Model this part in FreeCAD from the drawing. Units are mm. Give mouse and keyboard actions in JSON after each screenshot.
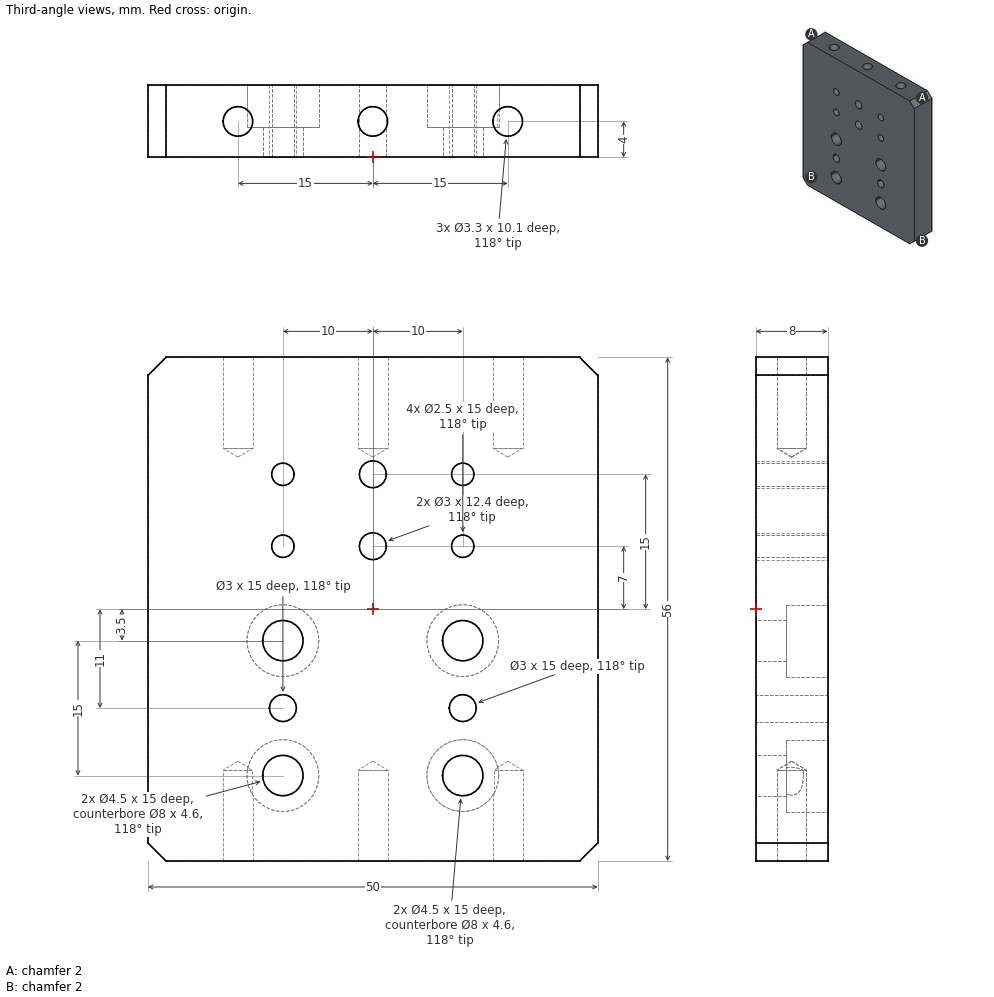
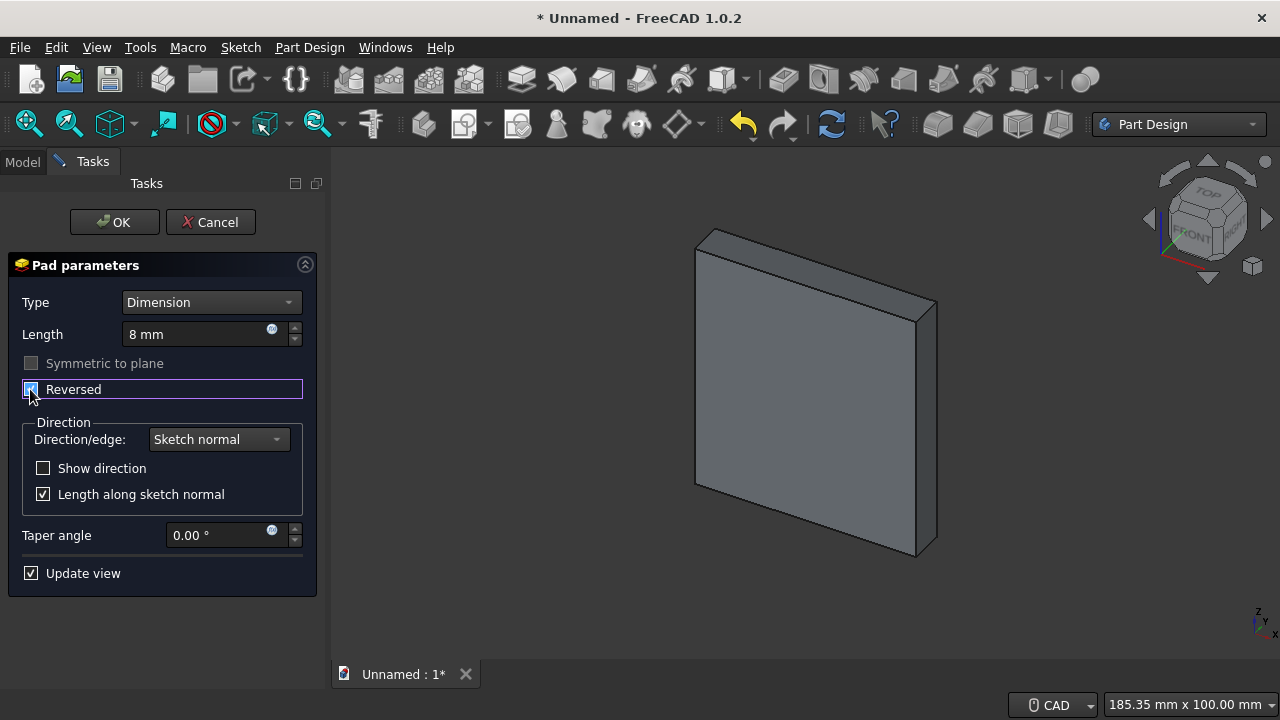
{"action": "left_click", "coordinate": [115, 222]}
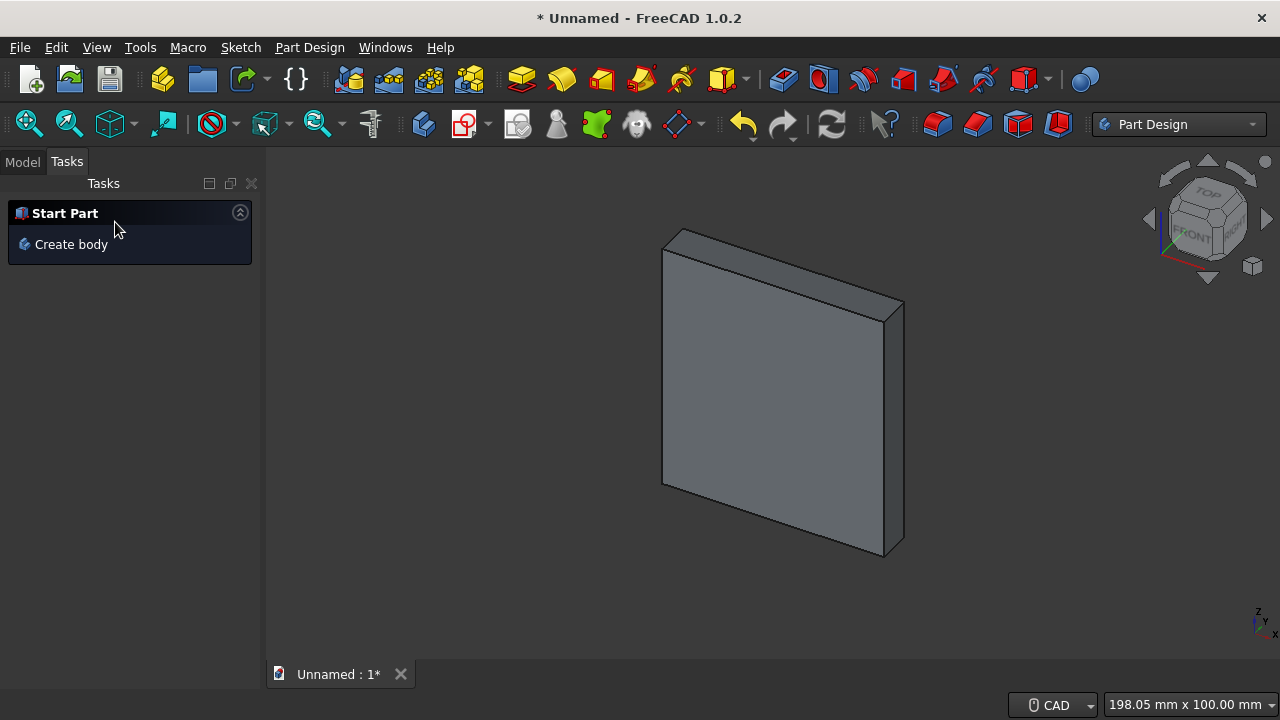
{"action": "left_click", "coordinate": [847, 295]}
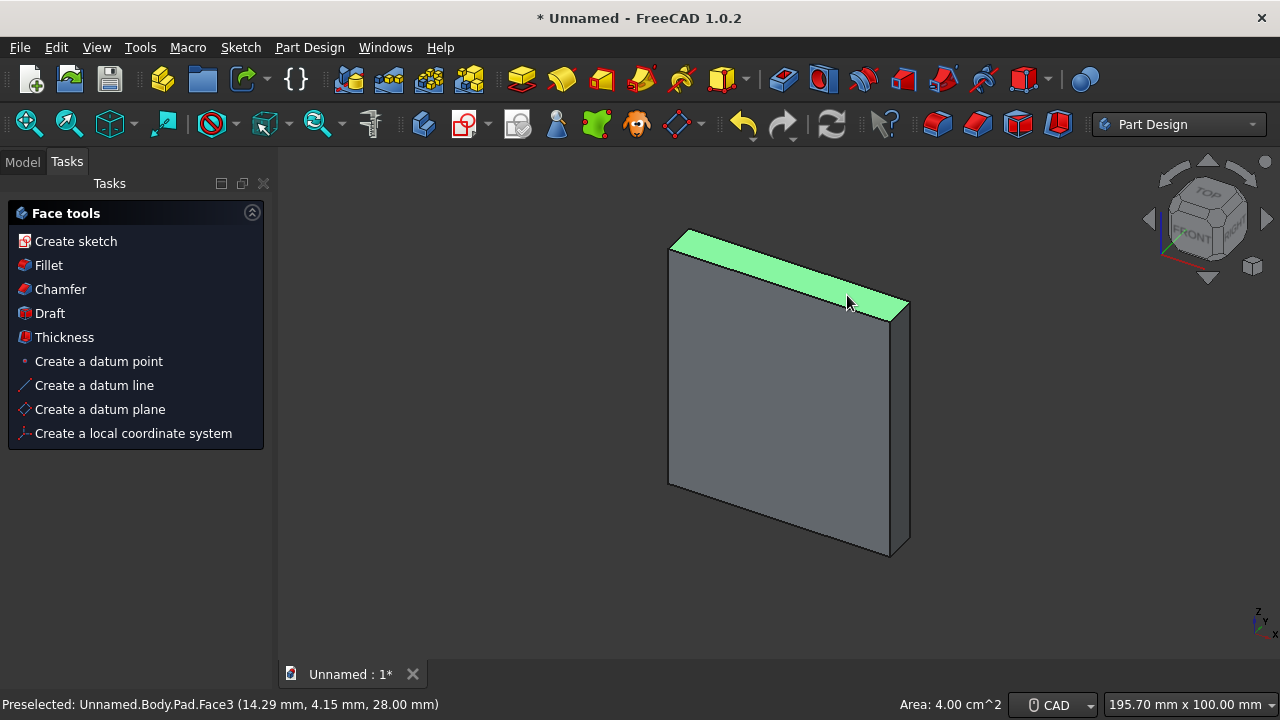
{"action": "left_click", "coordinate": [464, 124]}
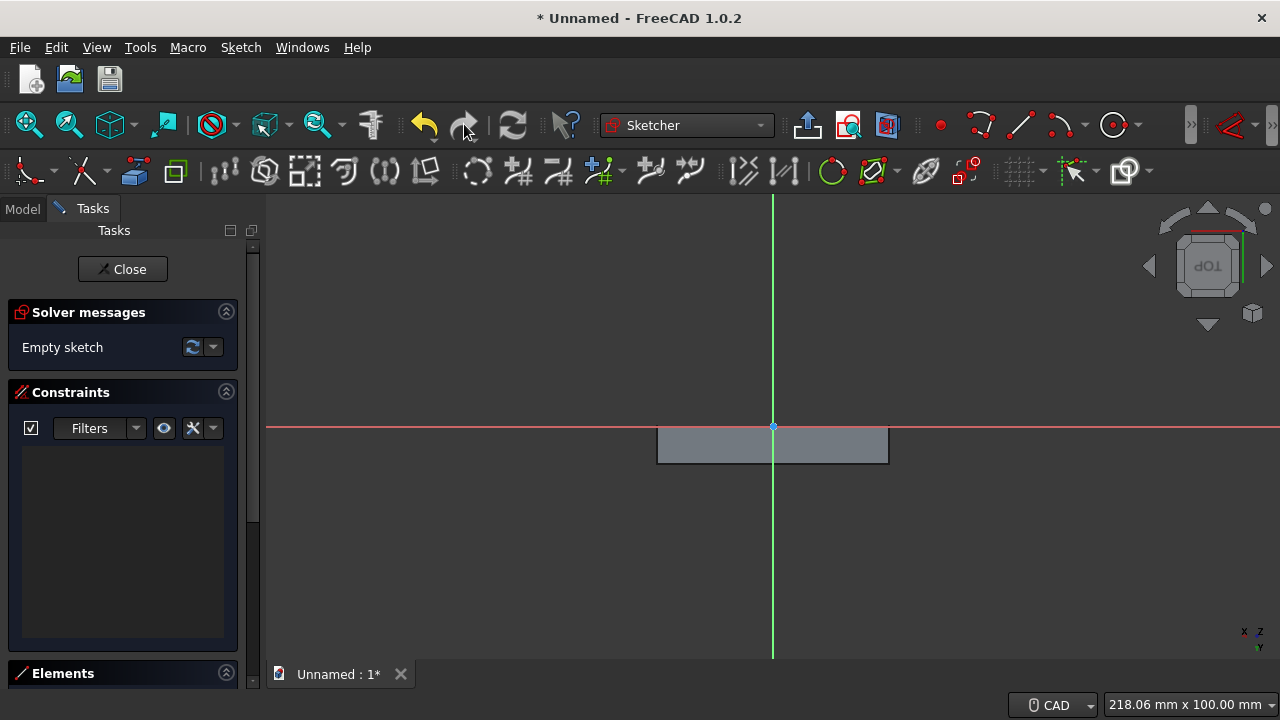
{"action": "scroll", "coordinate": [795, 444], "scroll_direction": "up", "scroll_amount": 7}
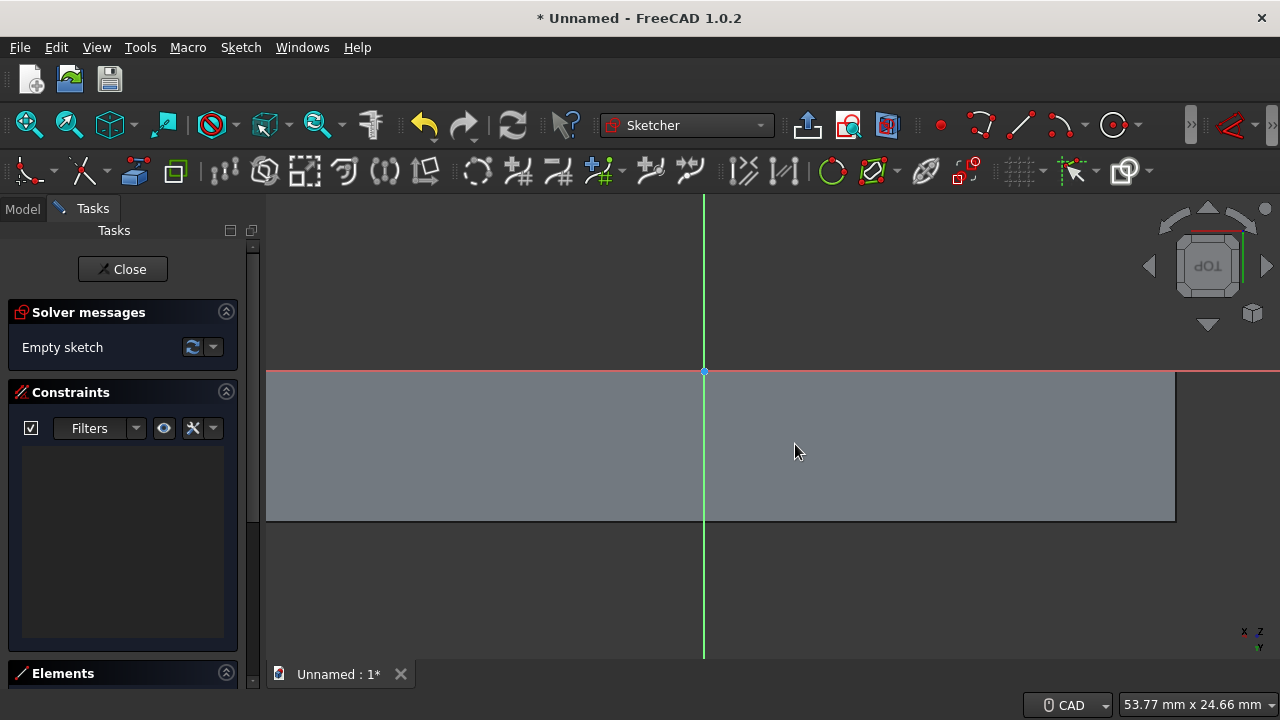
{"action": "left_click", "coordinate": [1114, 126]}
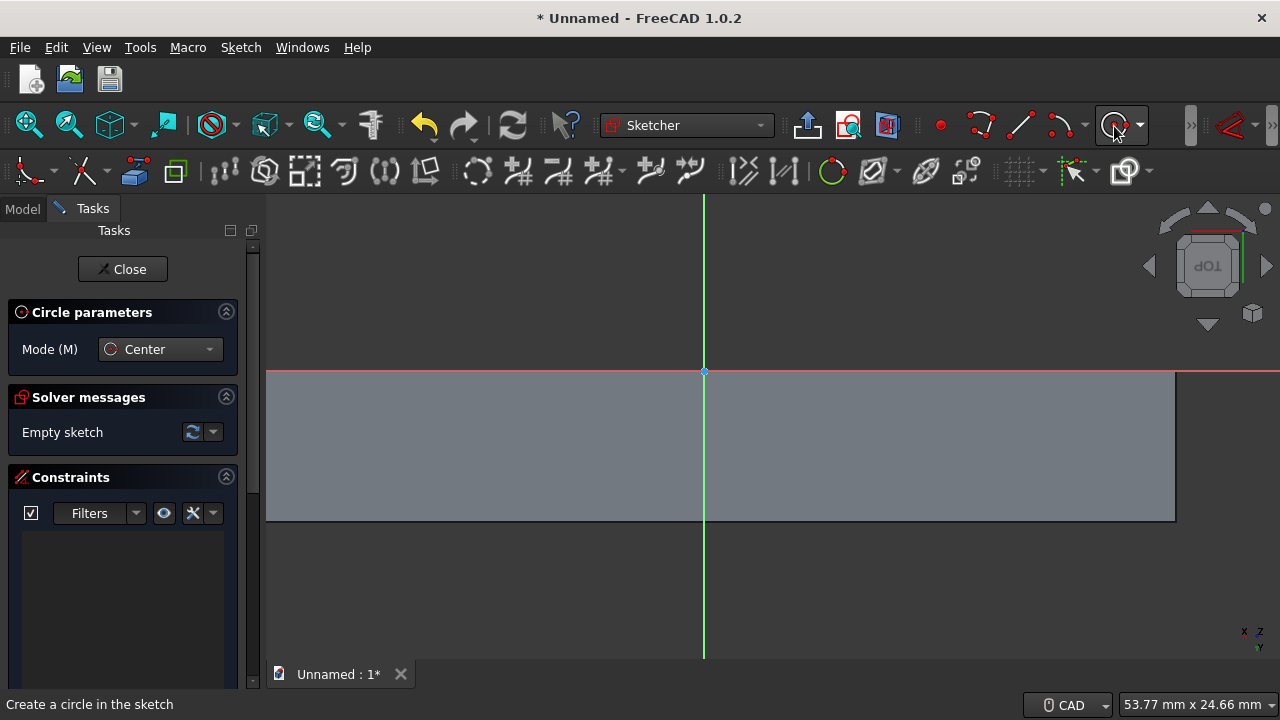
{"action": "left_click", "coordinate": [421, 447]}
{"action": "mouse_move", "coordinate": [443, 425]}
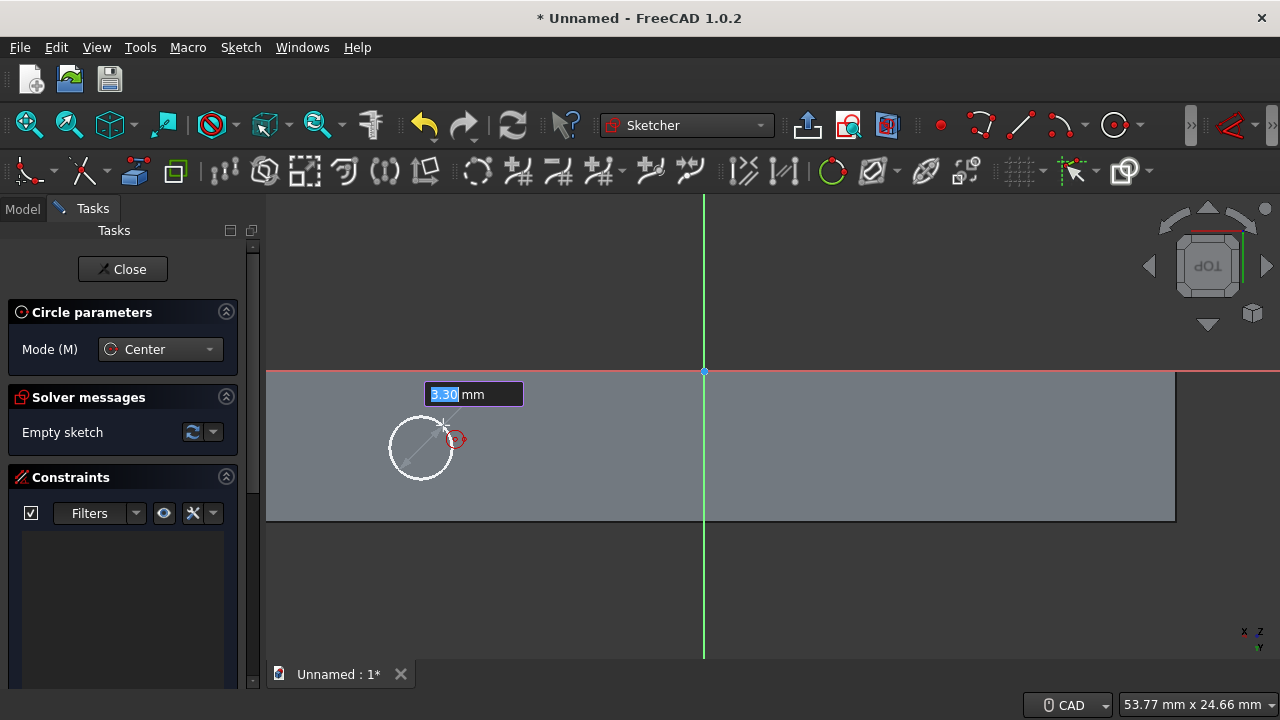
{"action": "type", "text": "3.3"}
{"action": "key", "text": "Return"}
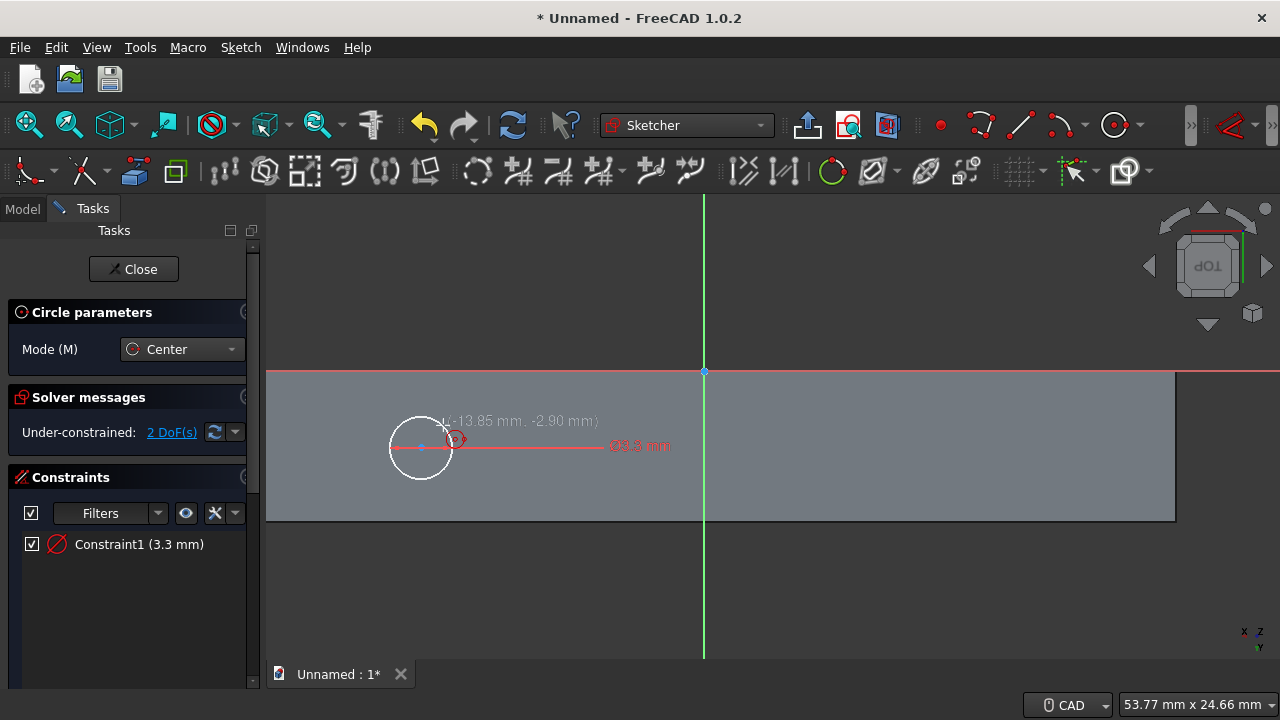
{"action": "left_click", "coordinate": [704, 447]}
{"action": "mouse_move", "coordinate": [726, 425]}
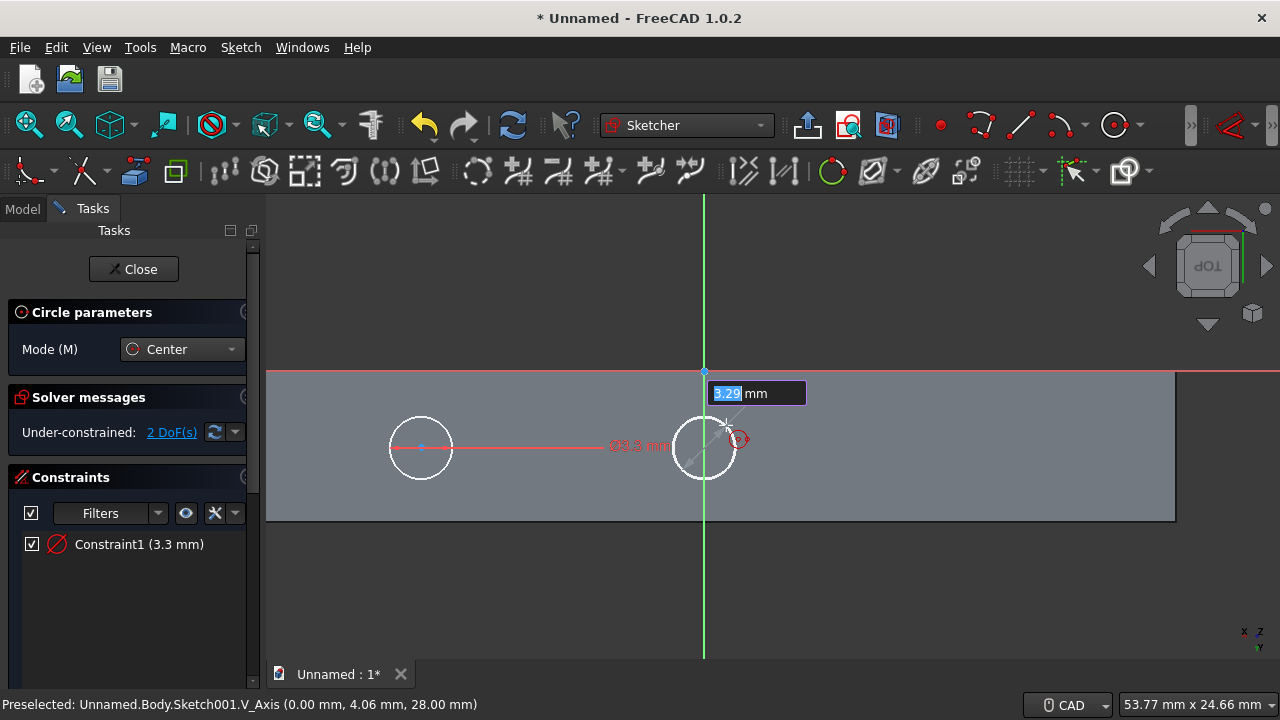
{"action": "type", "text": "3.3"}
{"action": "key", "text": "Return"}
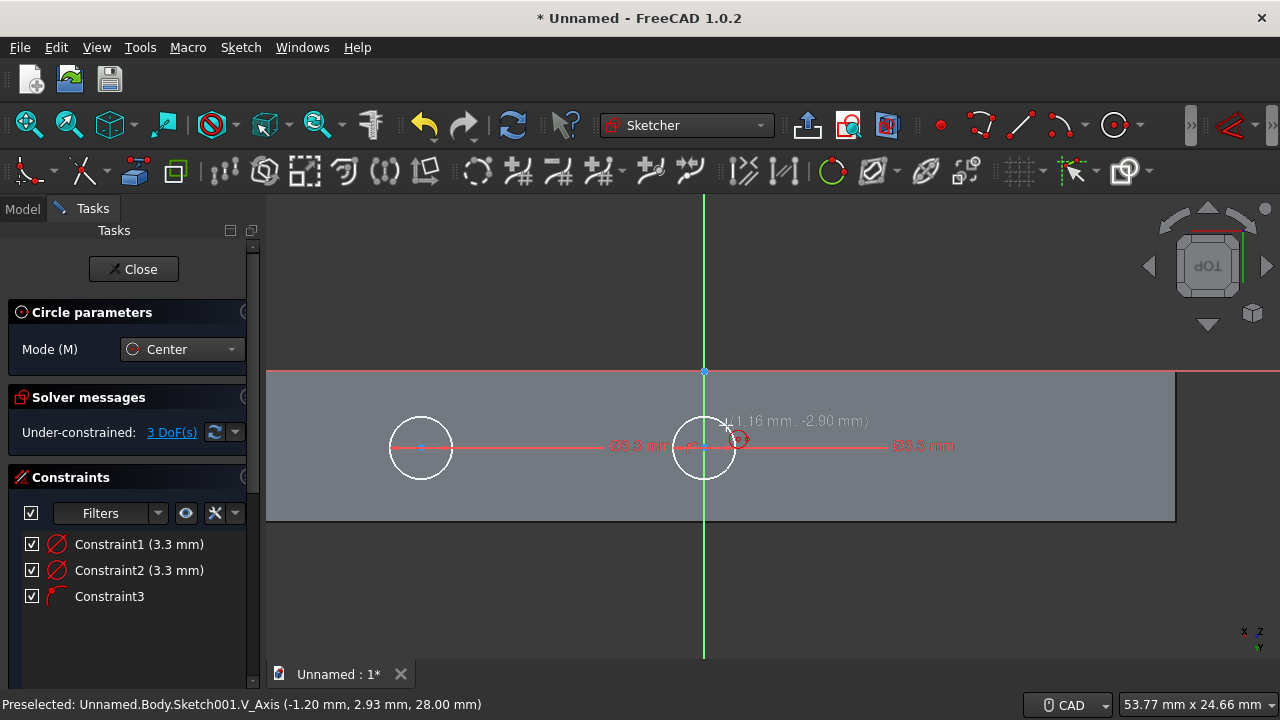
{"action": "left_click", "coordinate": [987, 447]}
{"action": "mouse_move", "coordinate": [1009, 425]}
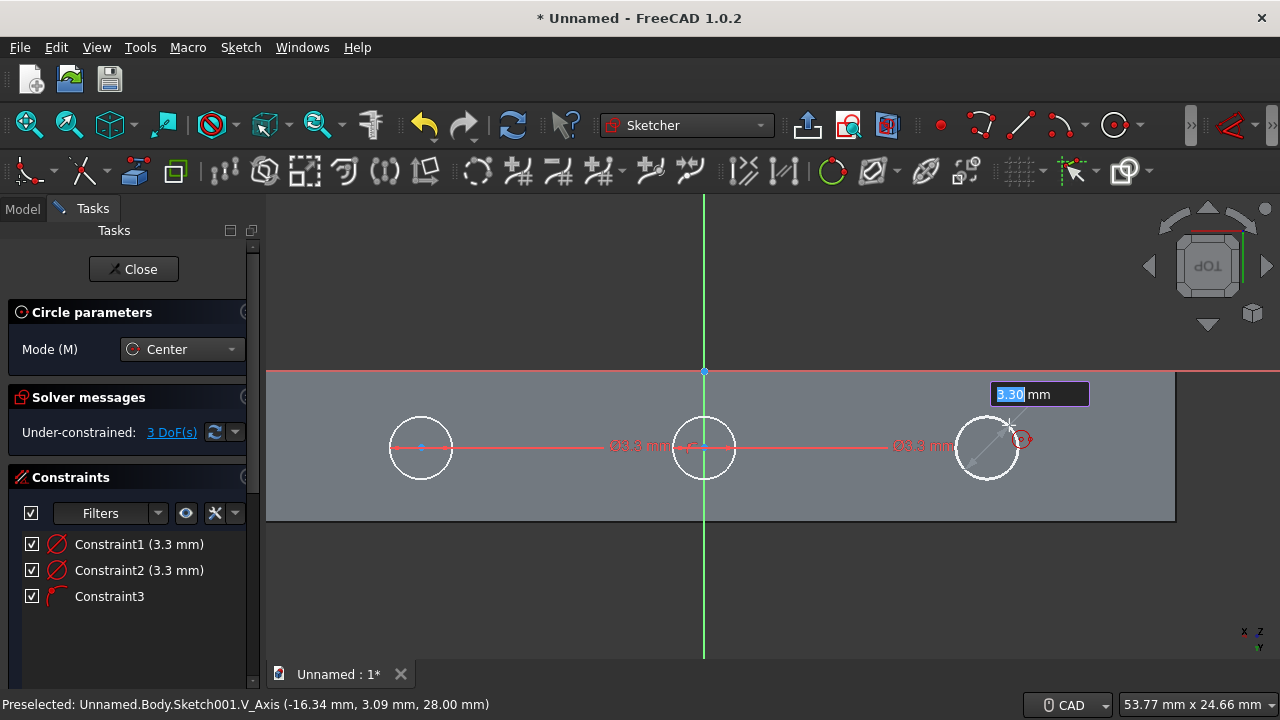
{"action": "type", "text": "3.3"}
{"action": "key", "text": "Return"}
{"action": "key", "text": "Escape"}